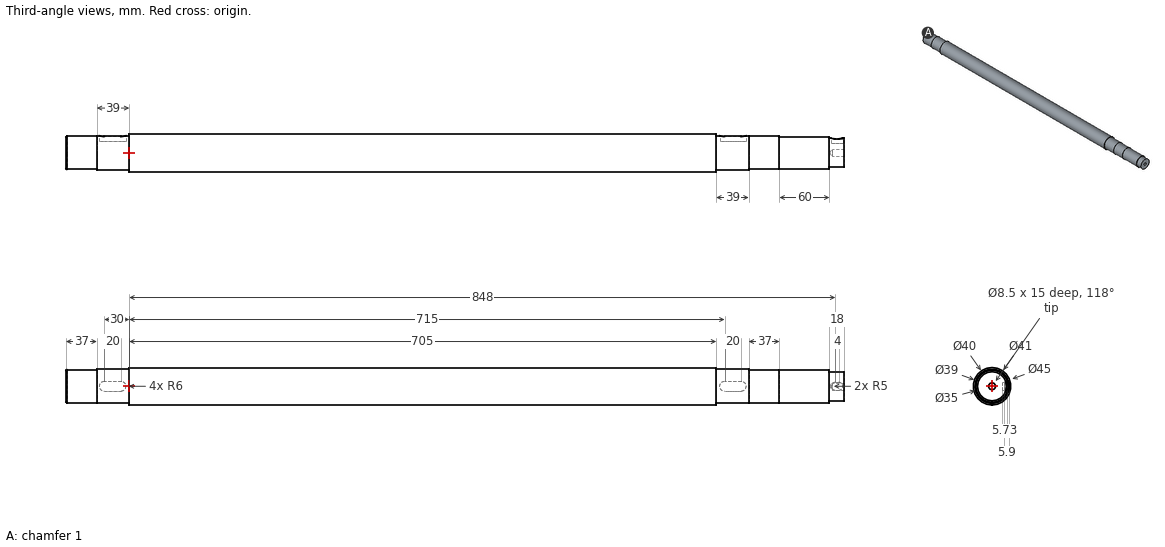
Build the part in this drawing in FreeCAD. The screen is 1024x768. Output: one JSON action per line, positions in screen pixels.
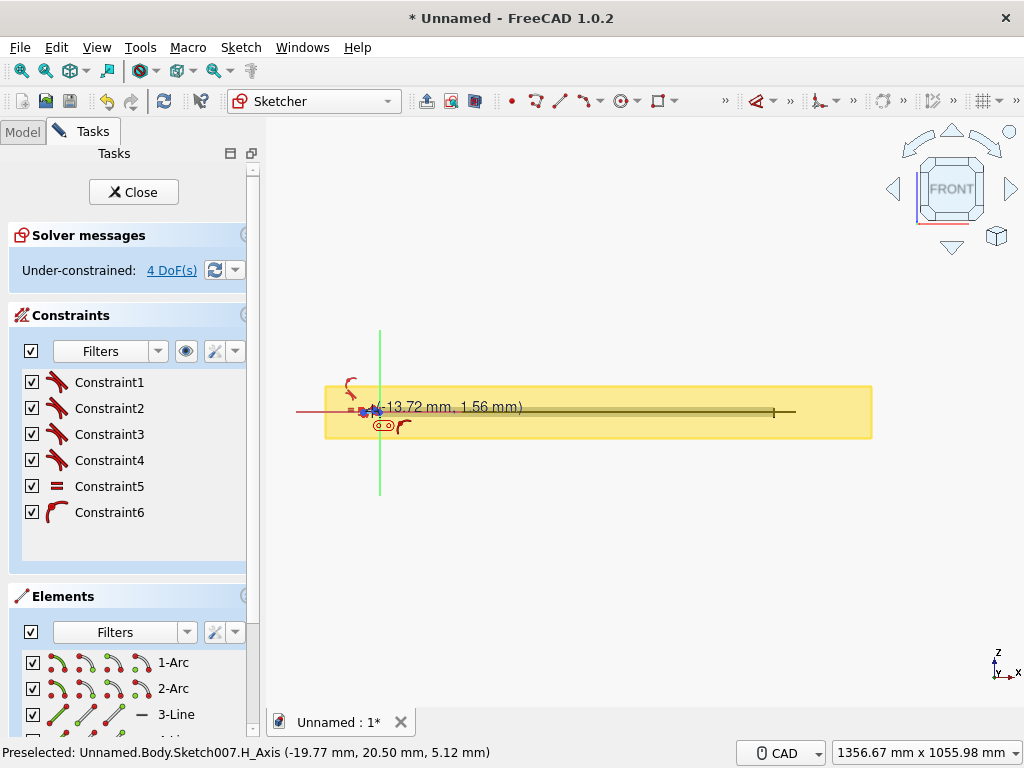
{"action": "scroll", "coordinate": [779, 412], "scroll_direction": "up", "scroll_amount": 10}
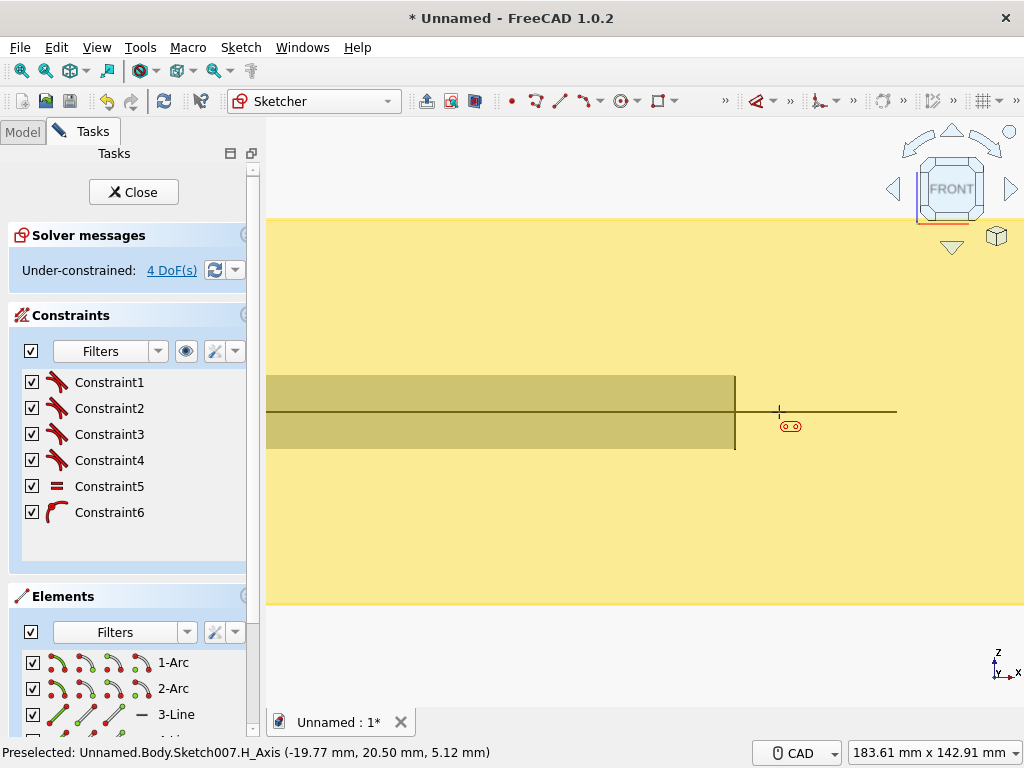
{"action": "scroll", "coordinate": [779, 412], "scroll_direction": "down", "scroll_amount": 10}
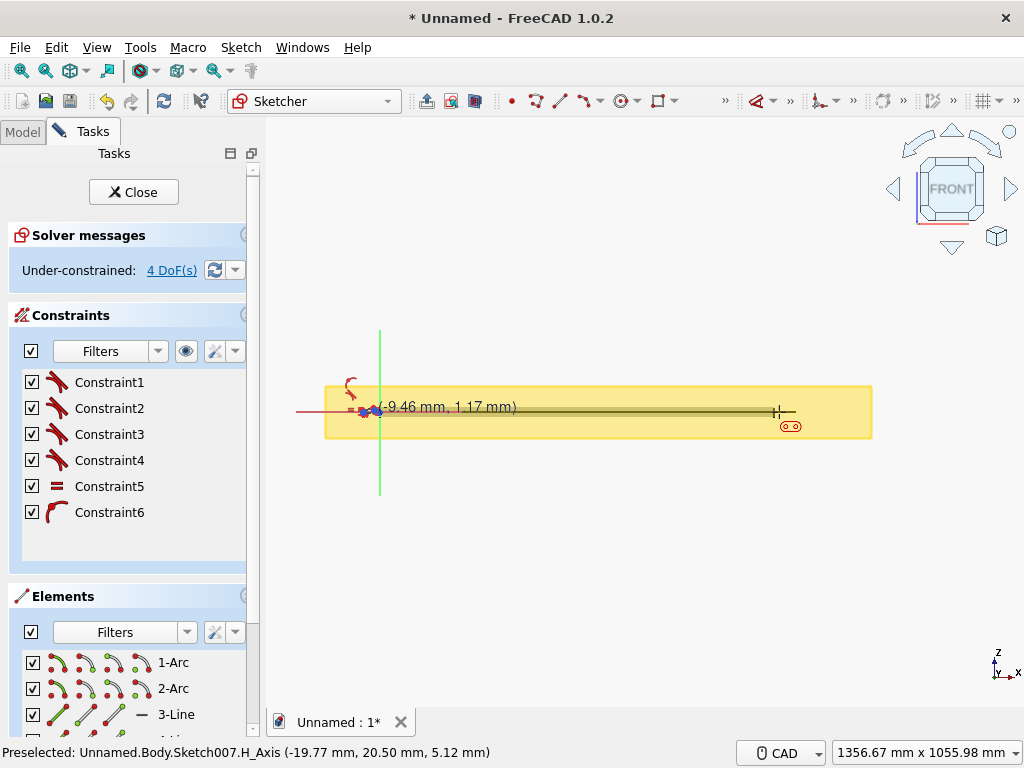
{"action": "left_click", "coordinate": [779, 412]}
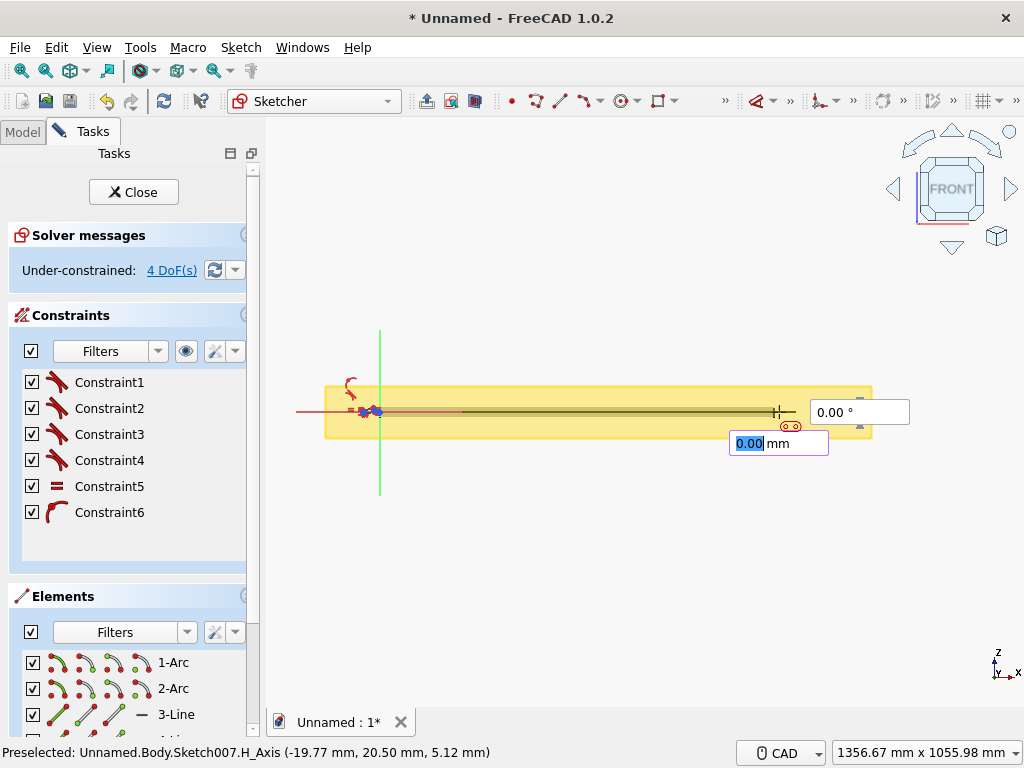
{"action": "scroll", "coordinate": [790, 412], "scroll_direction": "up", "scroll_amount": 2}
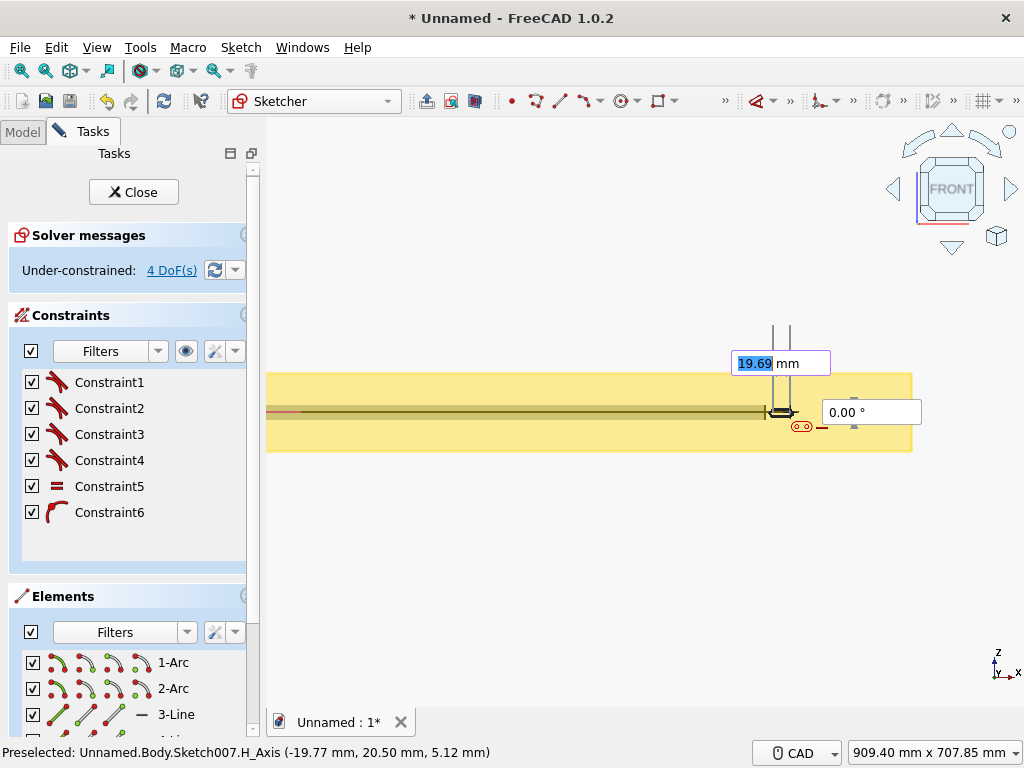
{"action": "left_click", "coordinate": [790, 403]}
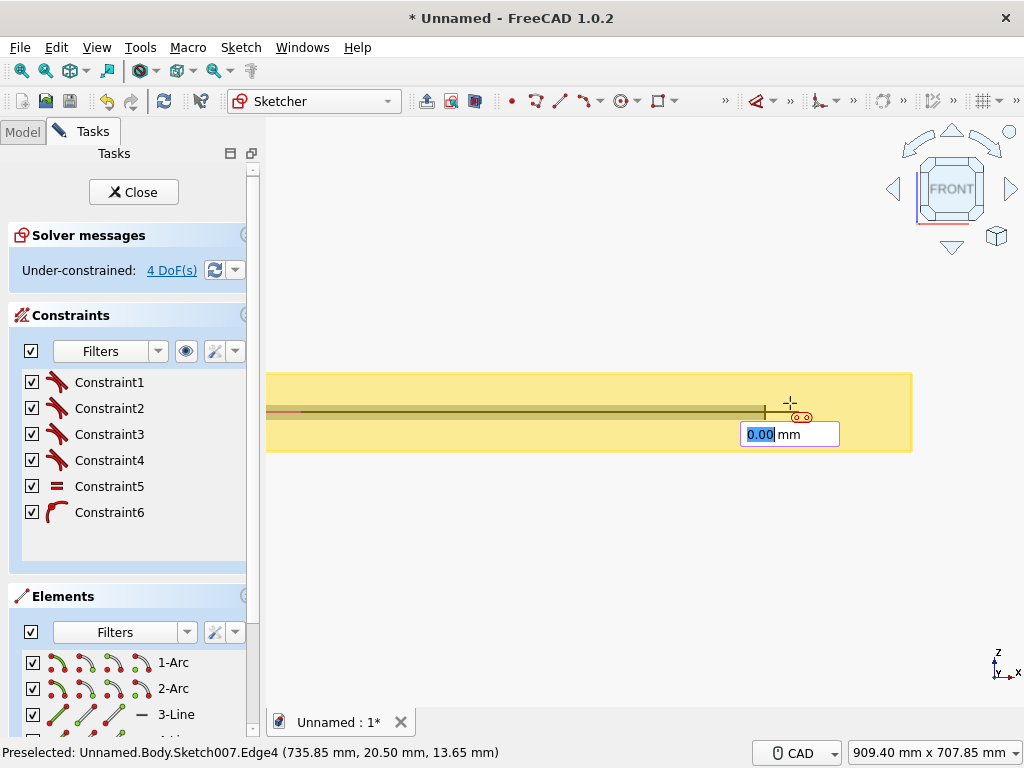
{"action": "scroll", "coordinate": [782, 417], "scroll_direction": "up", "scroll_amount": 6}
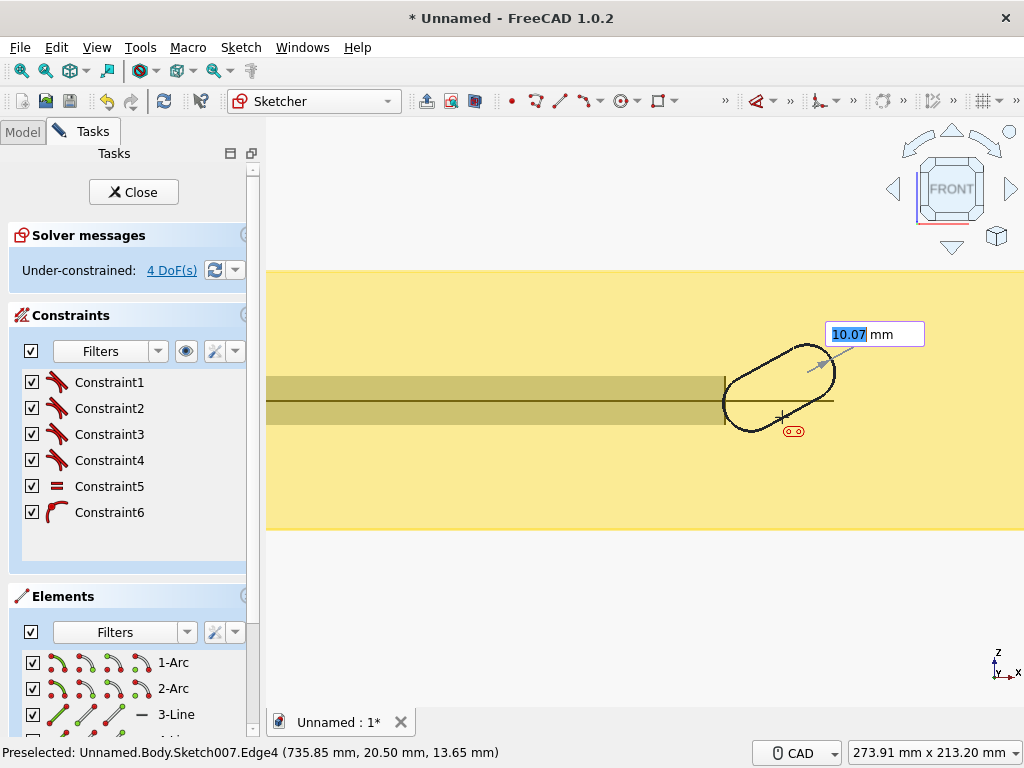
{"action": "left_click", "coordinate": [780, 417]}
{"action": "key", "text": "Escape"}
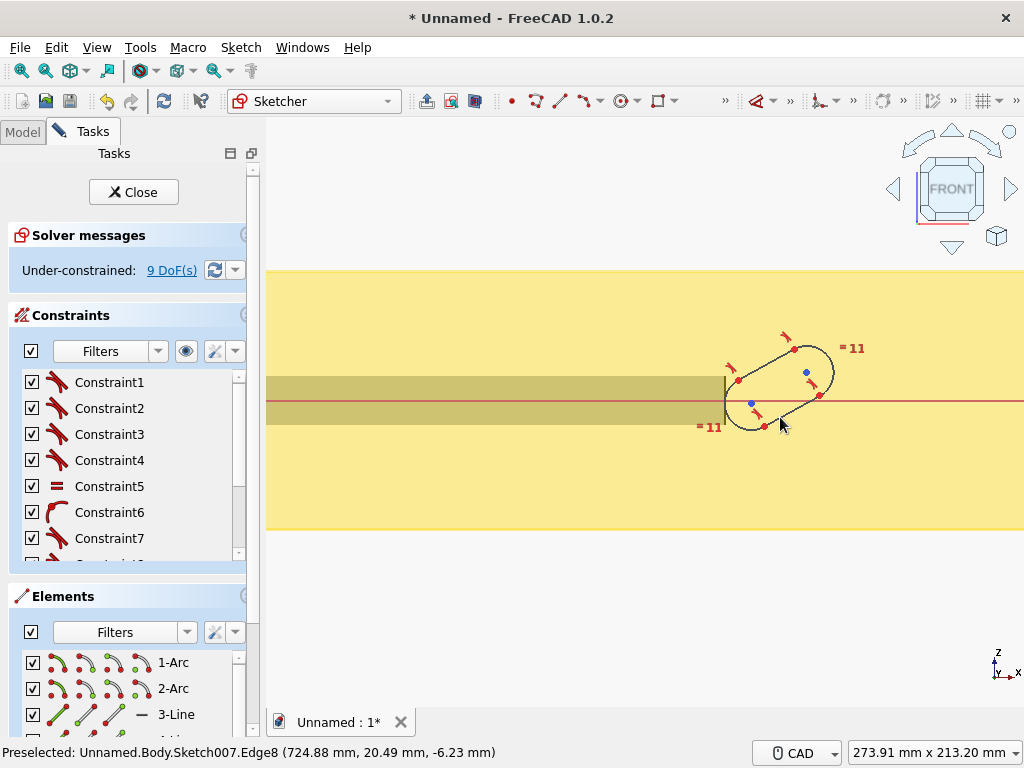
{"action": "scroll", "coordinate": [786, 415], "scroll_direction": "down", "scroll_amount": 8}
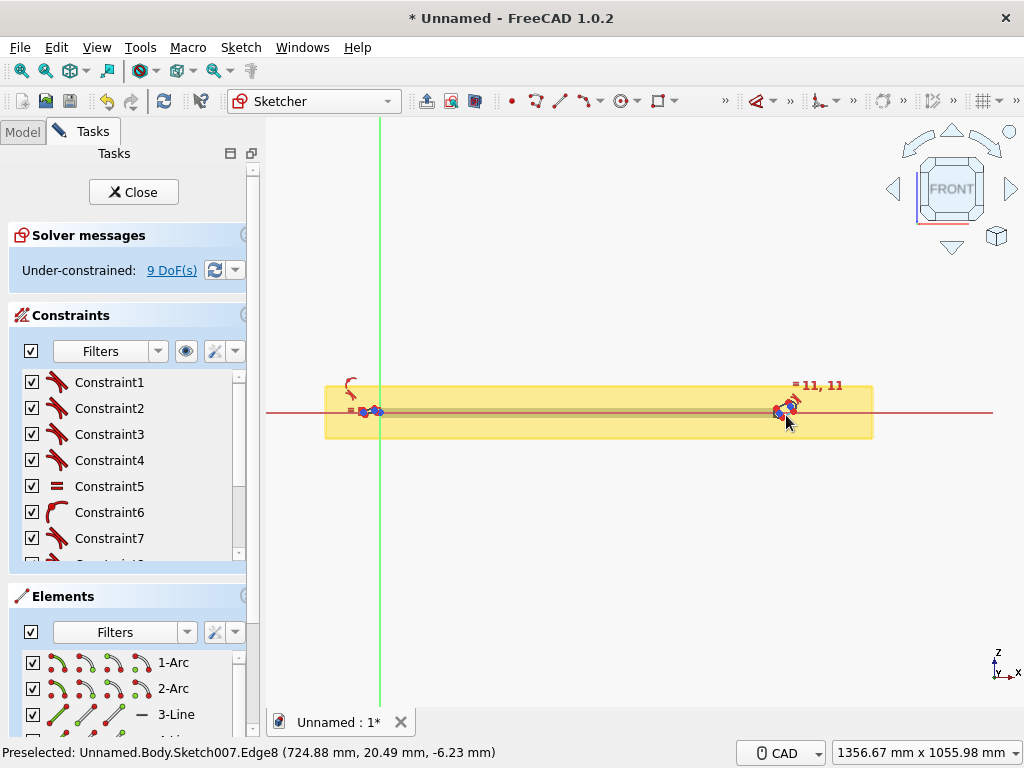
{"action": "scroll", "coordinate": [367, 410], "scroll_direction": "up", "scroll_amount": 9}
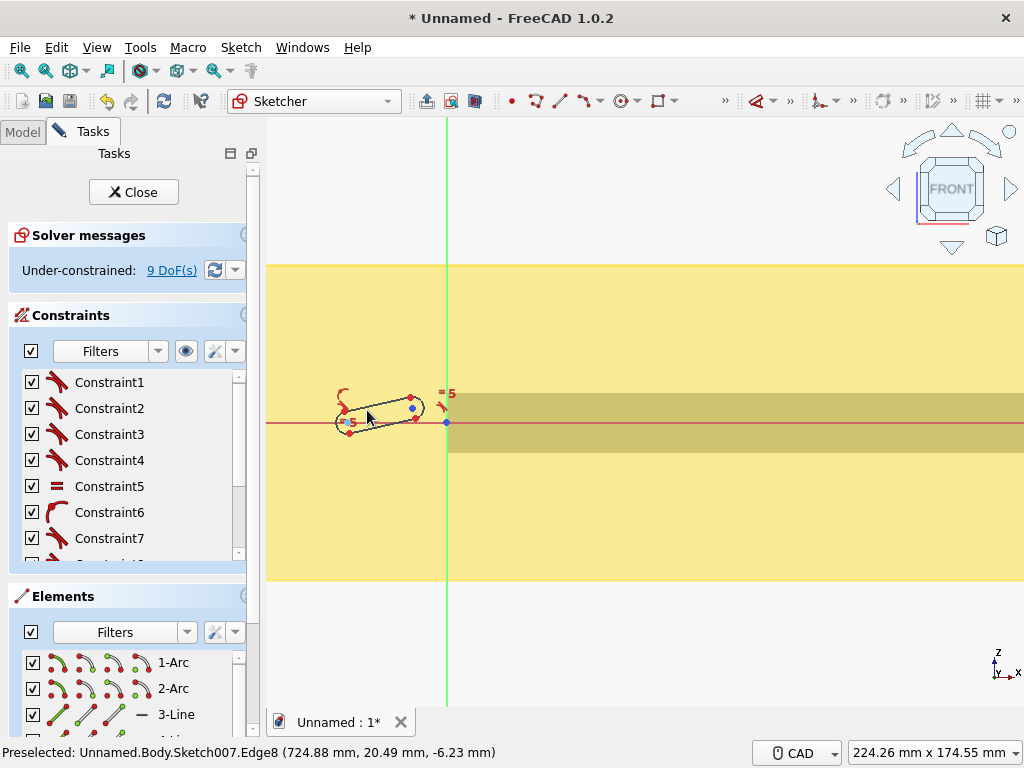
{"action": "left_click", "coordinate": [364, 408]}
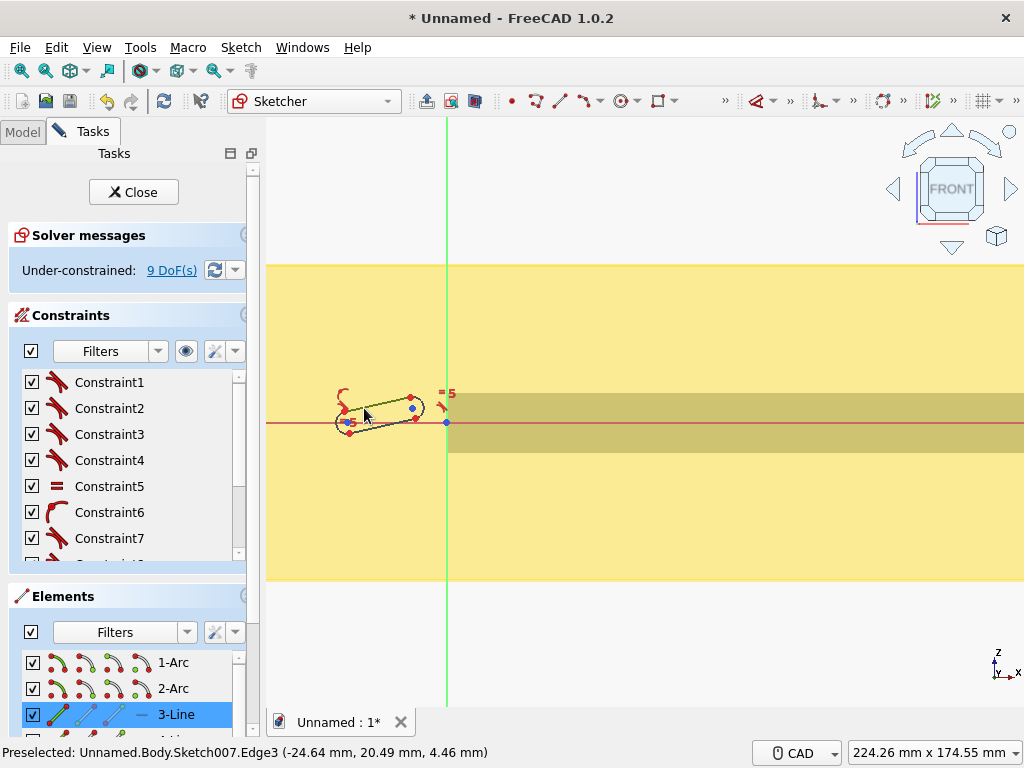
{"action": "key", "text": "h"}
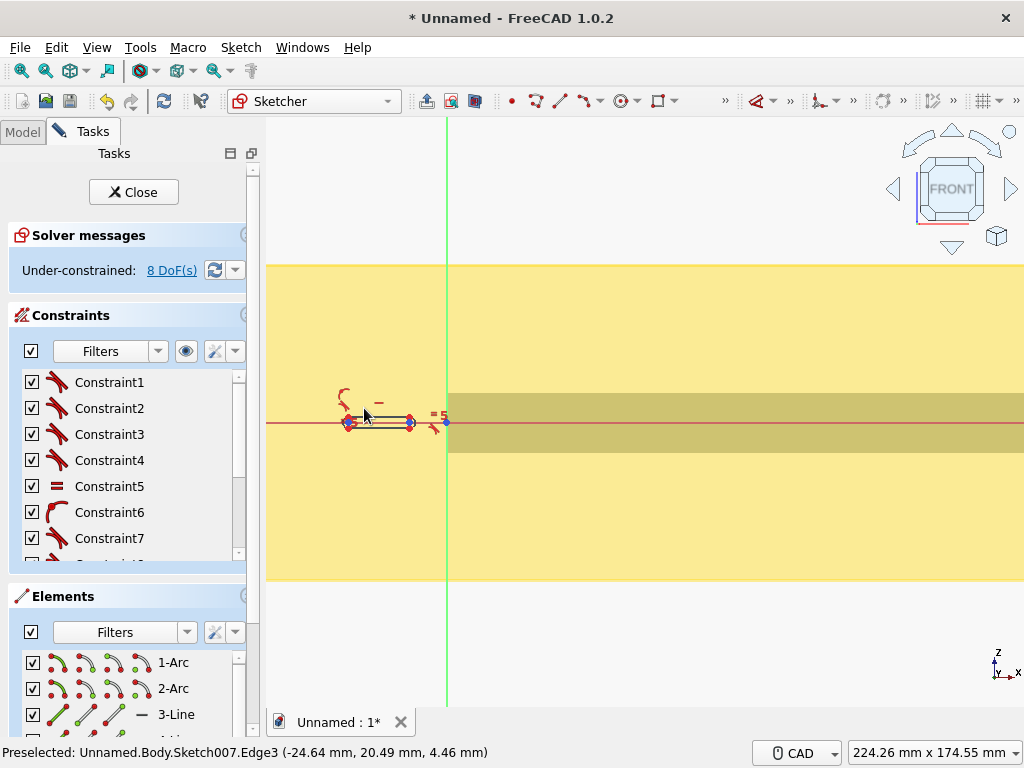
{"action": "scroll", "coordinate": [366, 410], "scroll_direction": "down", "scroll_amount": 9}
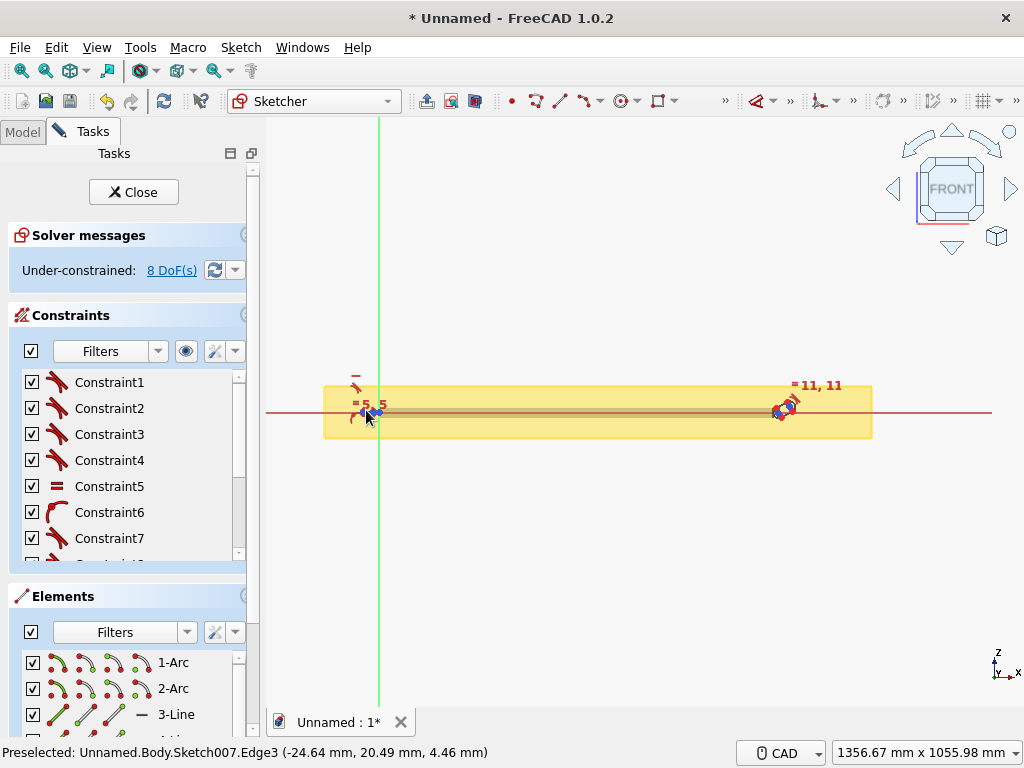
{"action": "scroll", "coordinate": [779, 406], "scroll_direction": "up", "scroll_amount": 7}